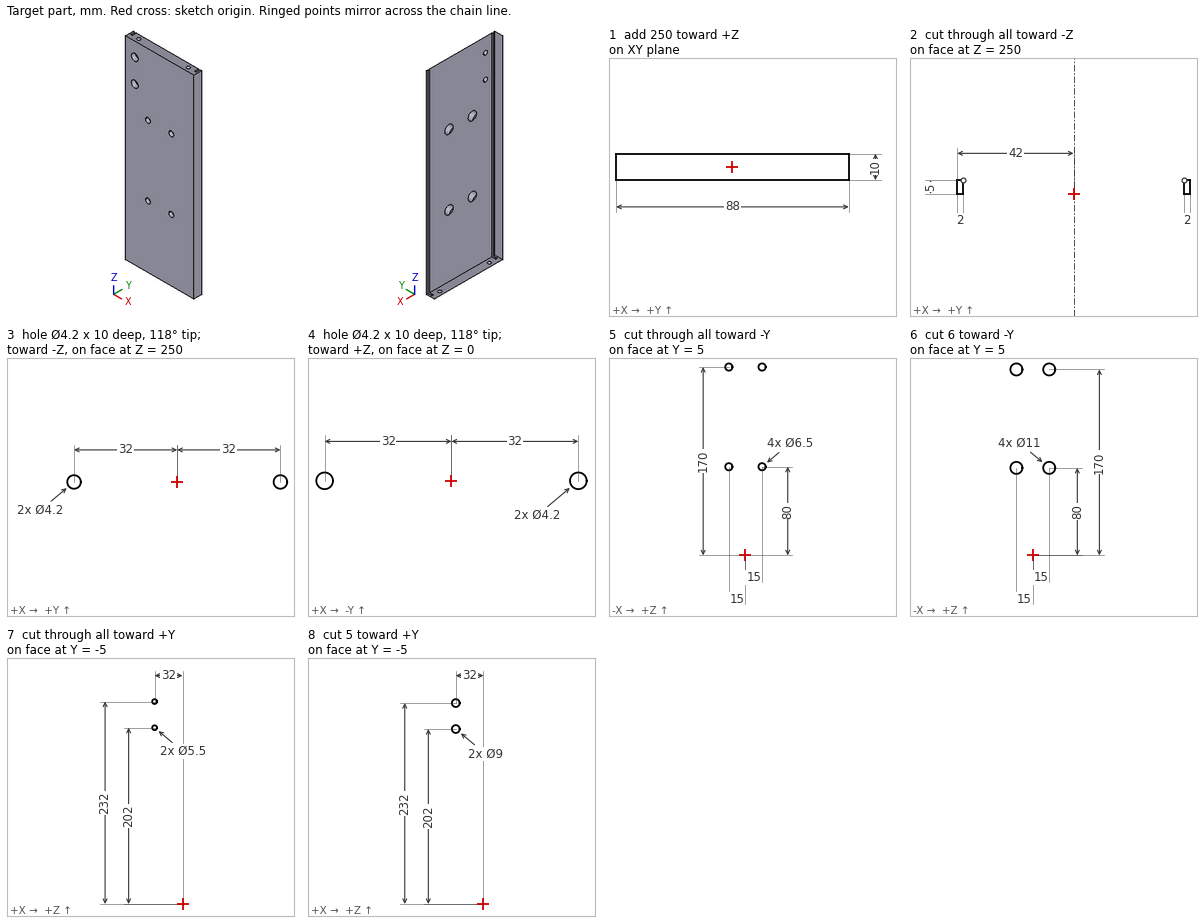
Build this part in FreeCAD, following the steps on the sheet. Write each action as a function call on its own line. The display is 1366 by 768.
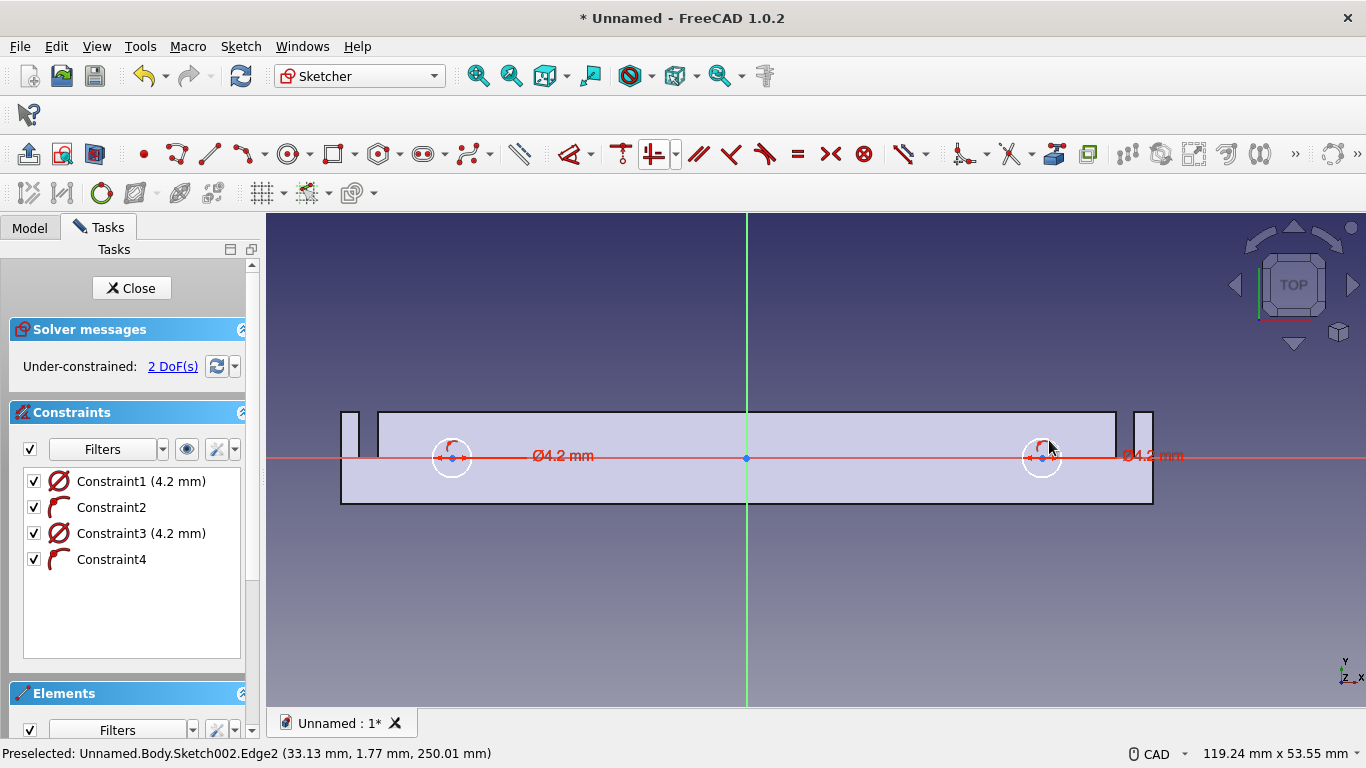
click(568, 154)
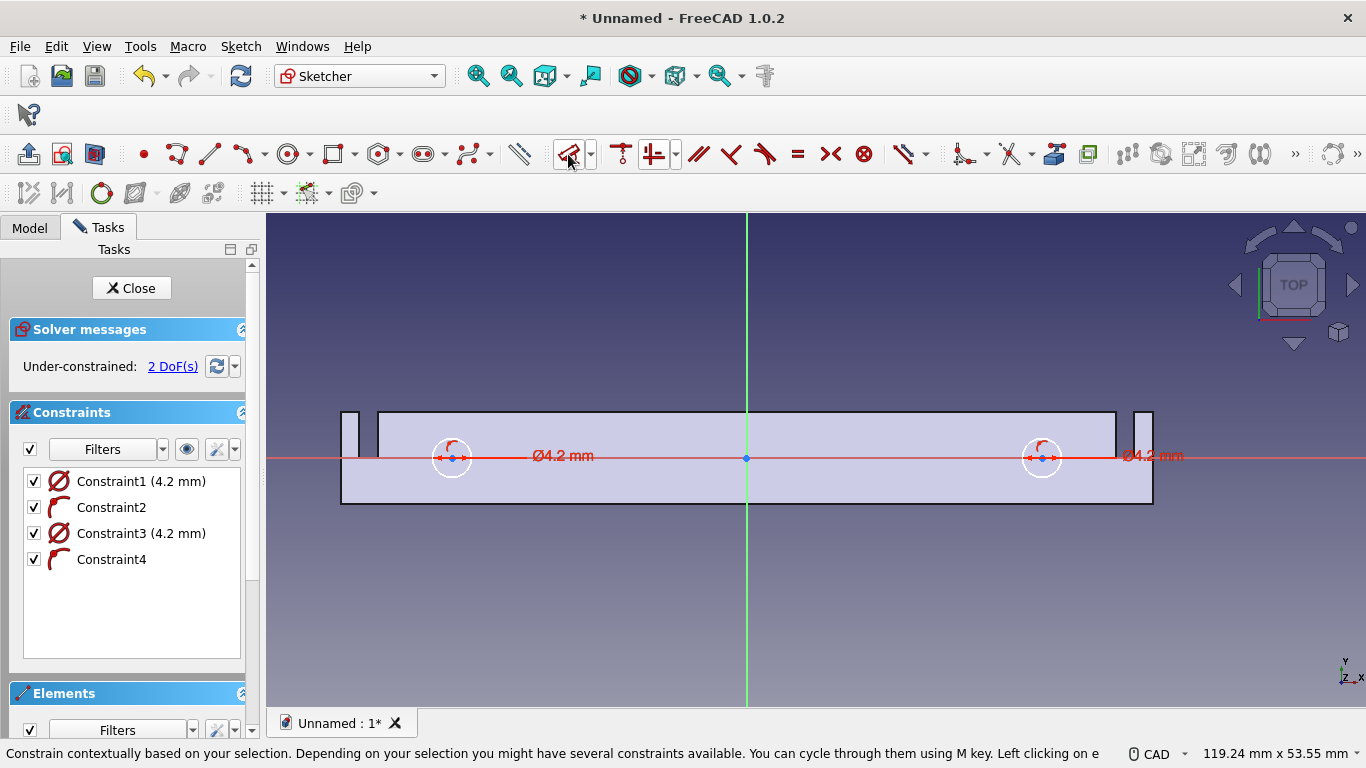
click(452, 458)
click(599, 492)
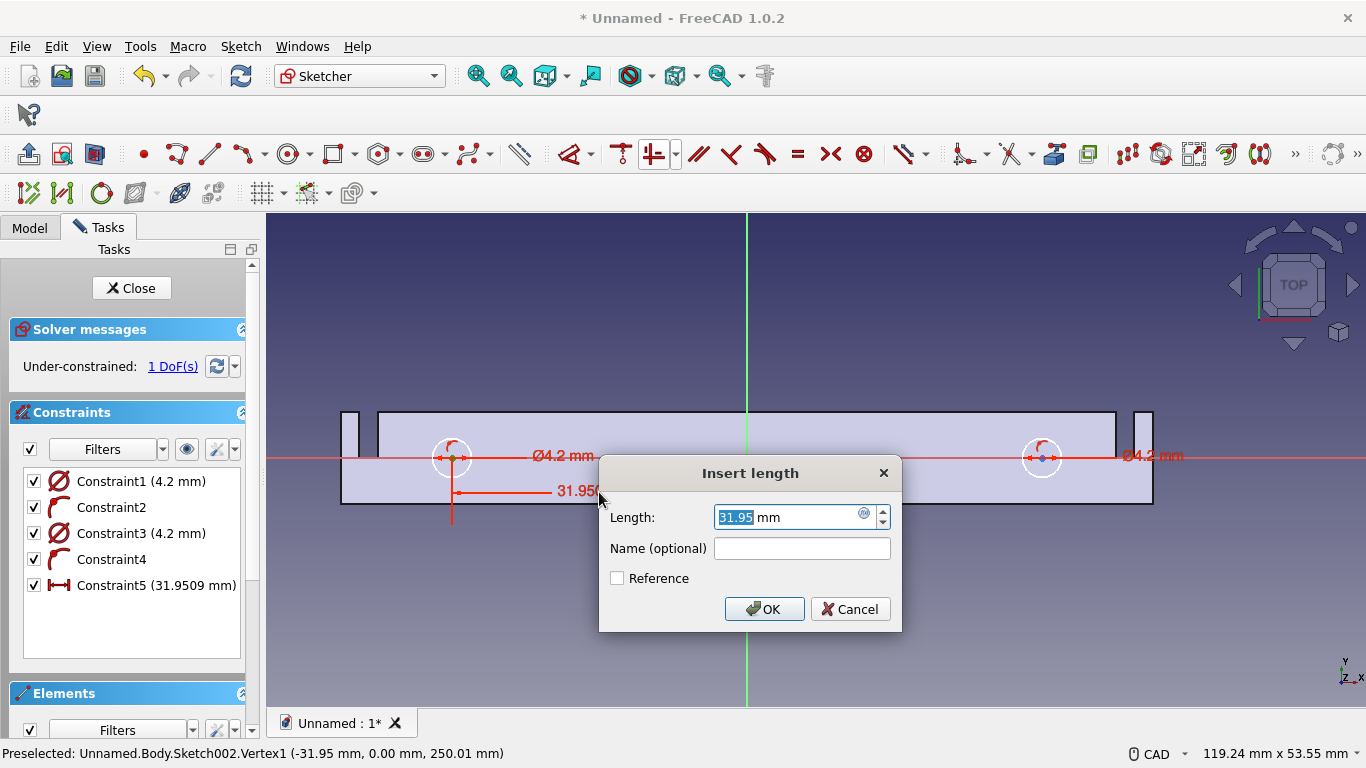
text(32)
key(Return)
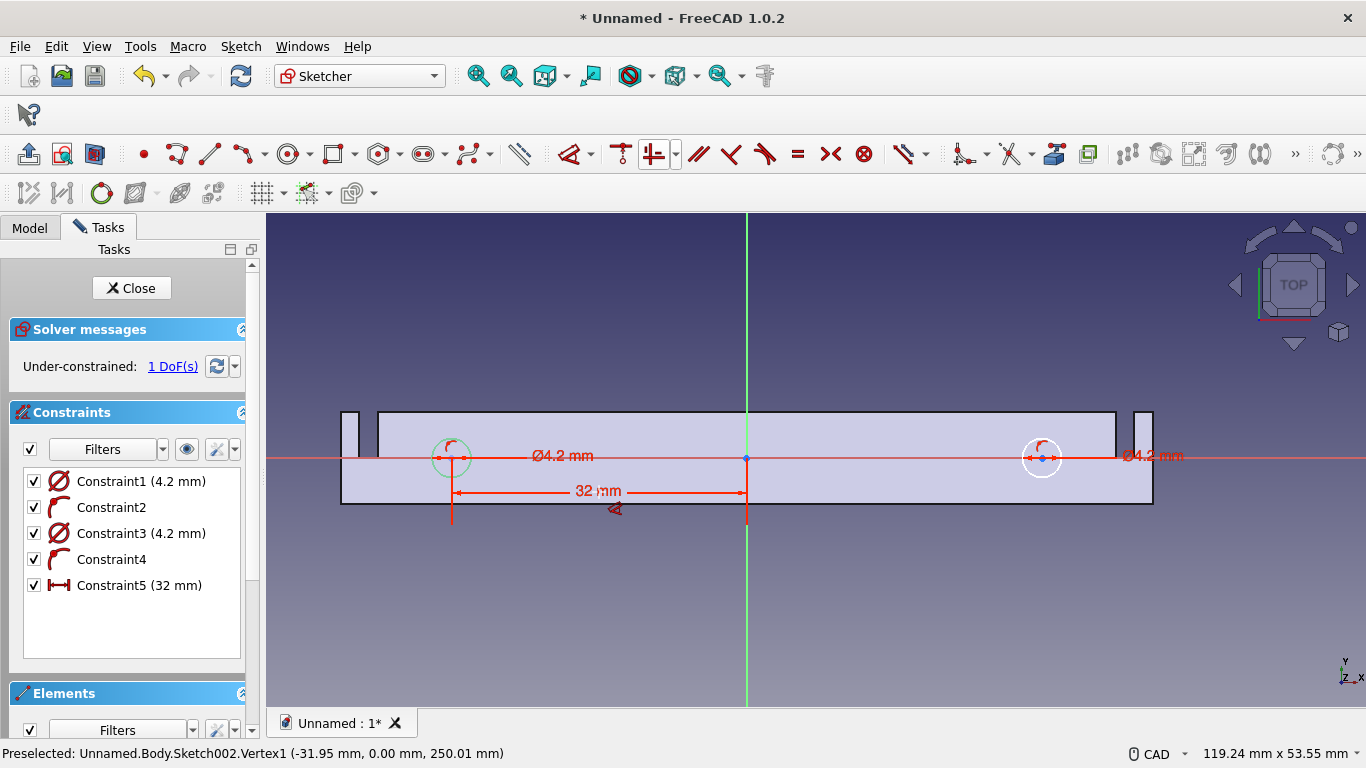
click(1042, 458)
click(894, 492)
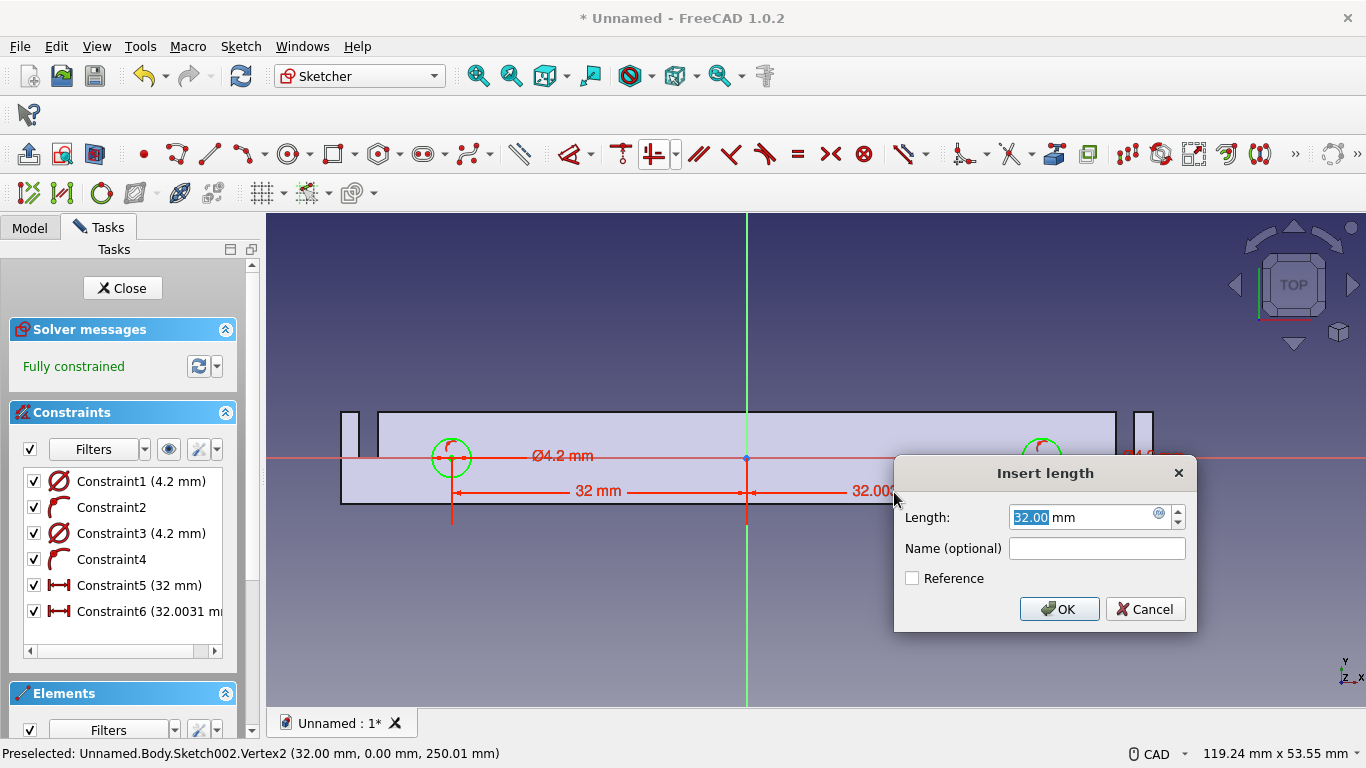
text(32)
key(Return)
key(Escape)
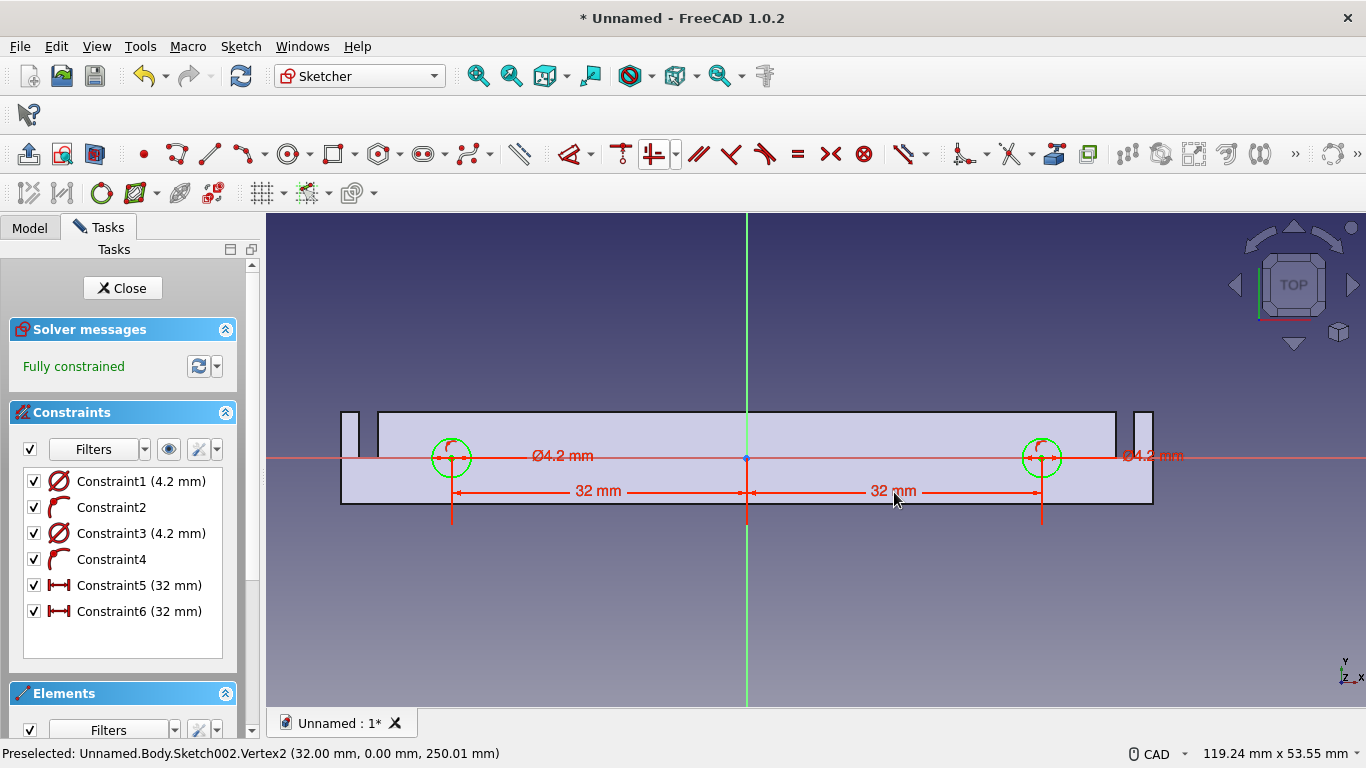
click(123, 288)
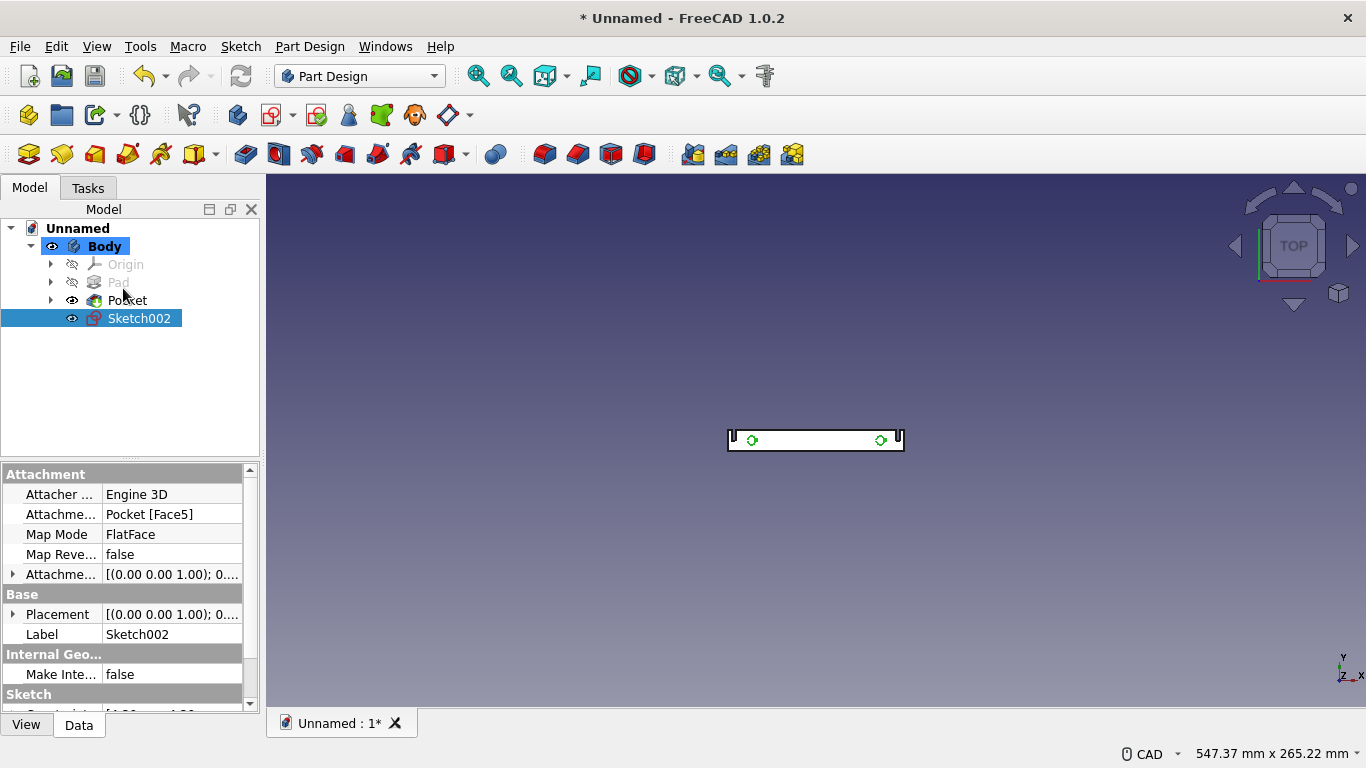
click(279, 154)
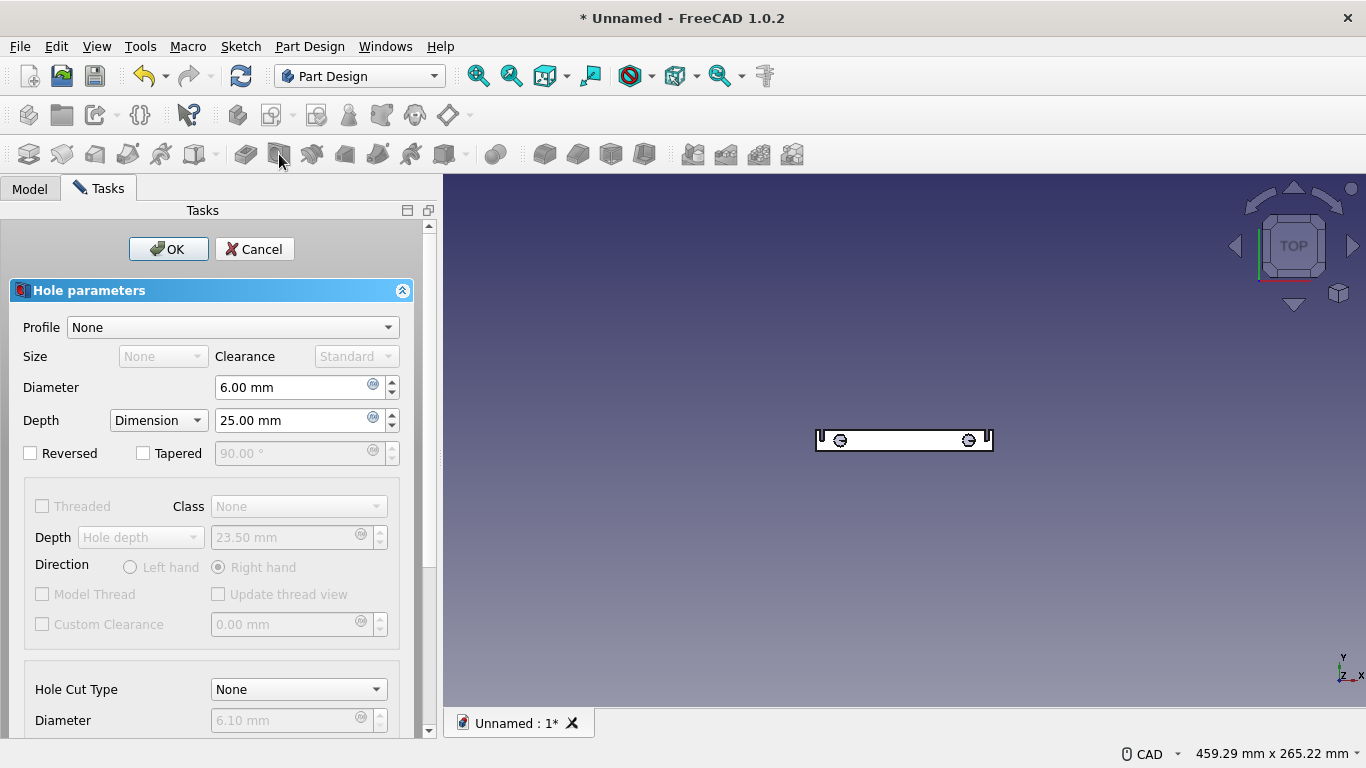
triple_click(300, 388)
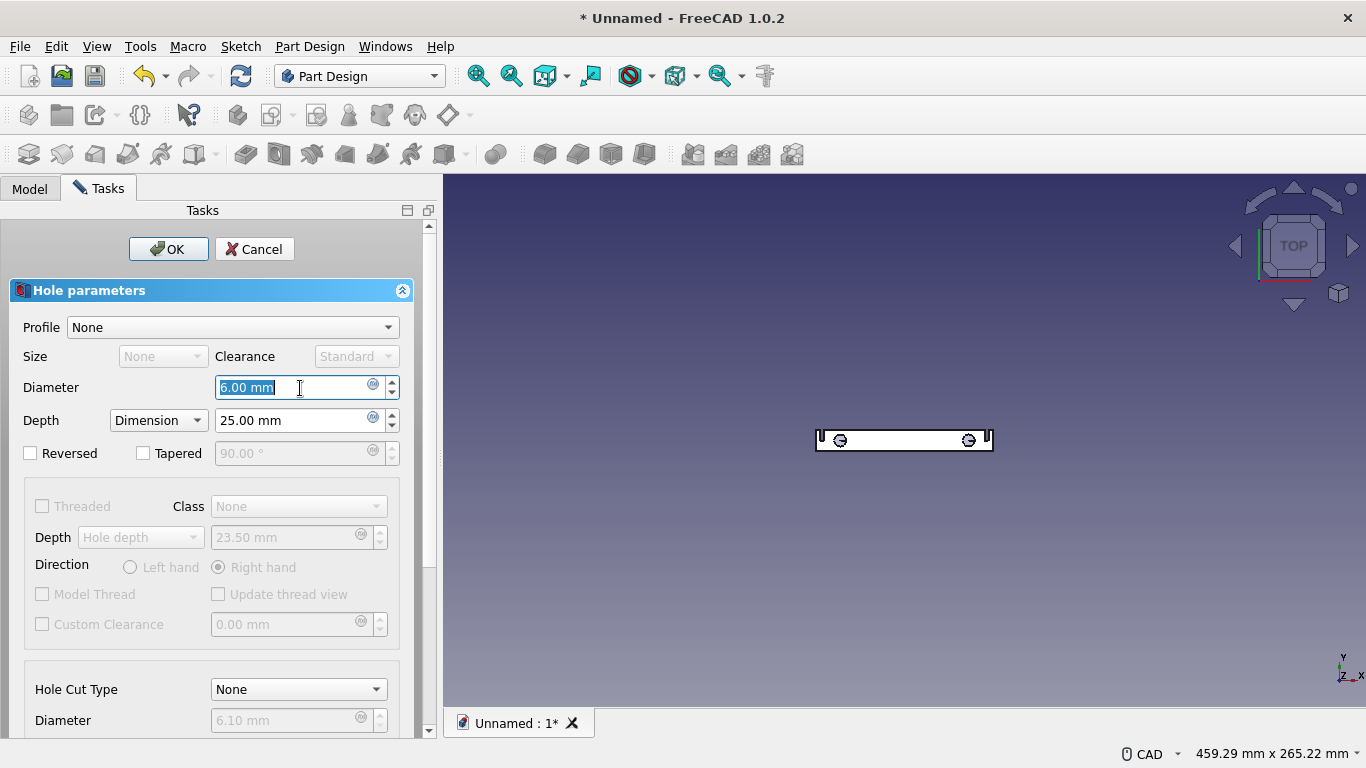
text(4.2)
key(Tab)